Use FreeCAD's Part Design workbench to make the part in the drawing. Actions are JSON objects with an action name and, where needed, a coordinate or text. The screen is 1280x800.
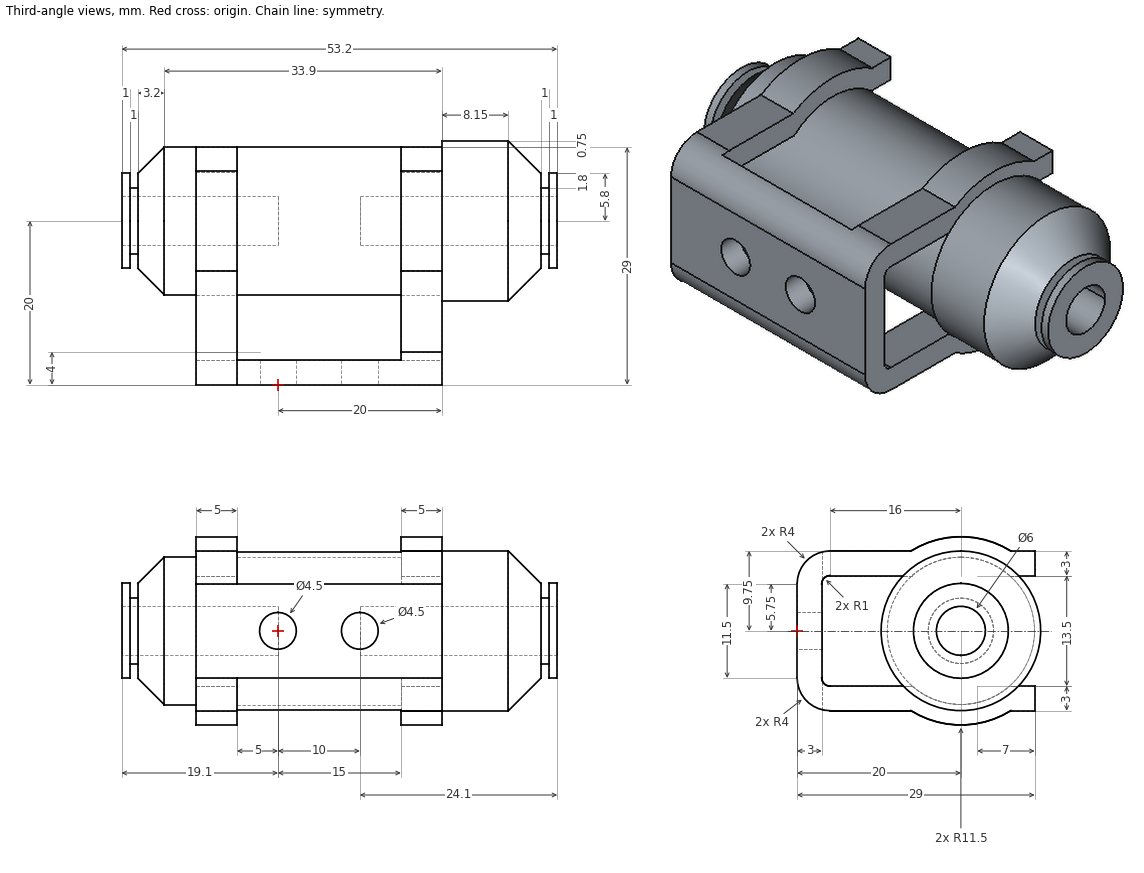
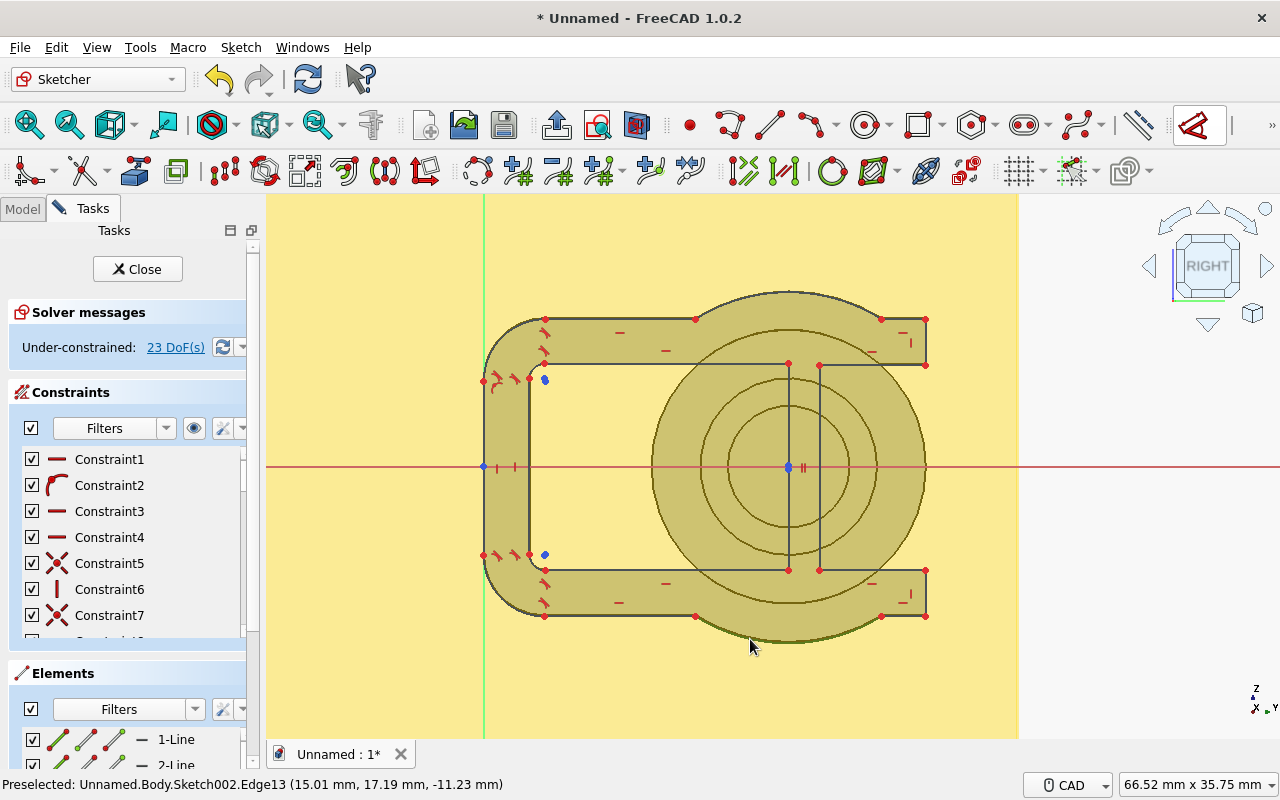
{"action": "left_click", "coordinate": [827, 297]}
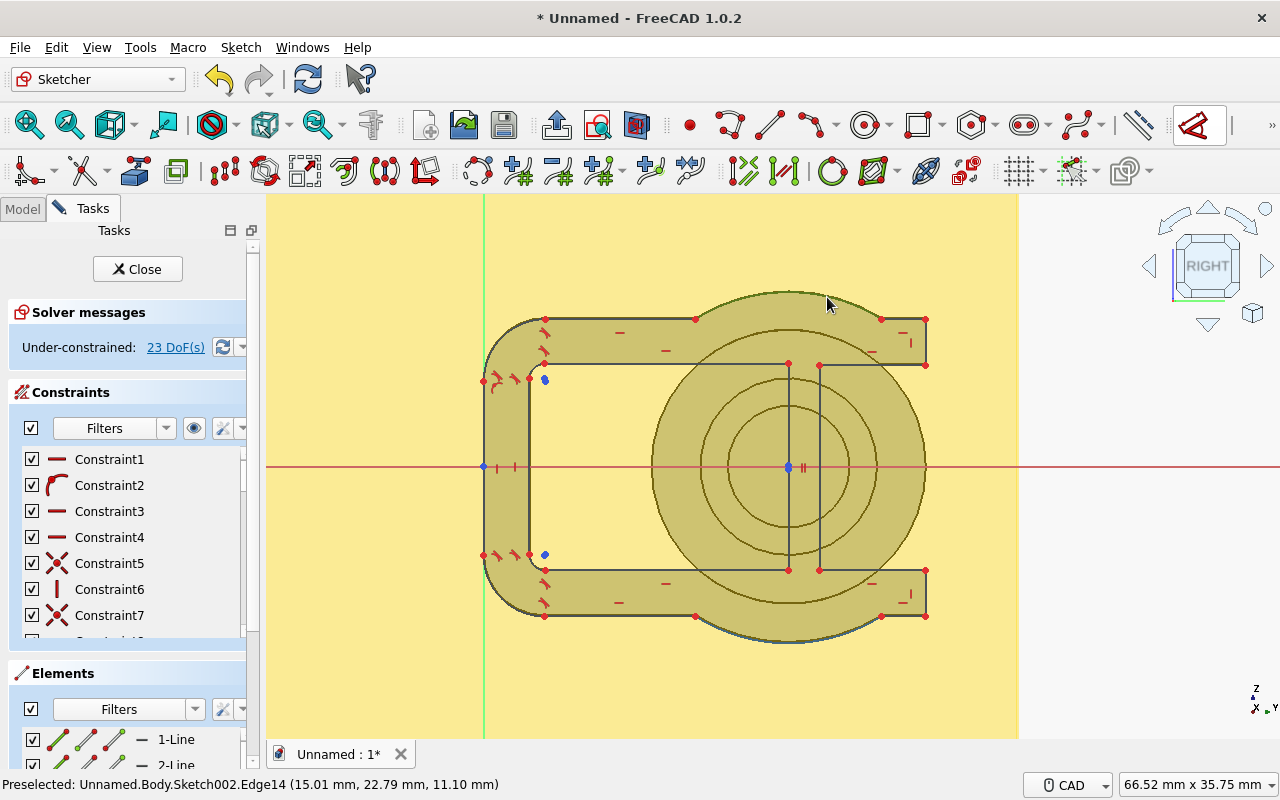
{"action": "key", "text": "c"}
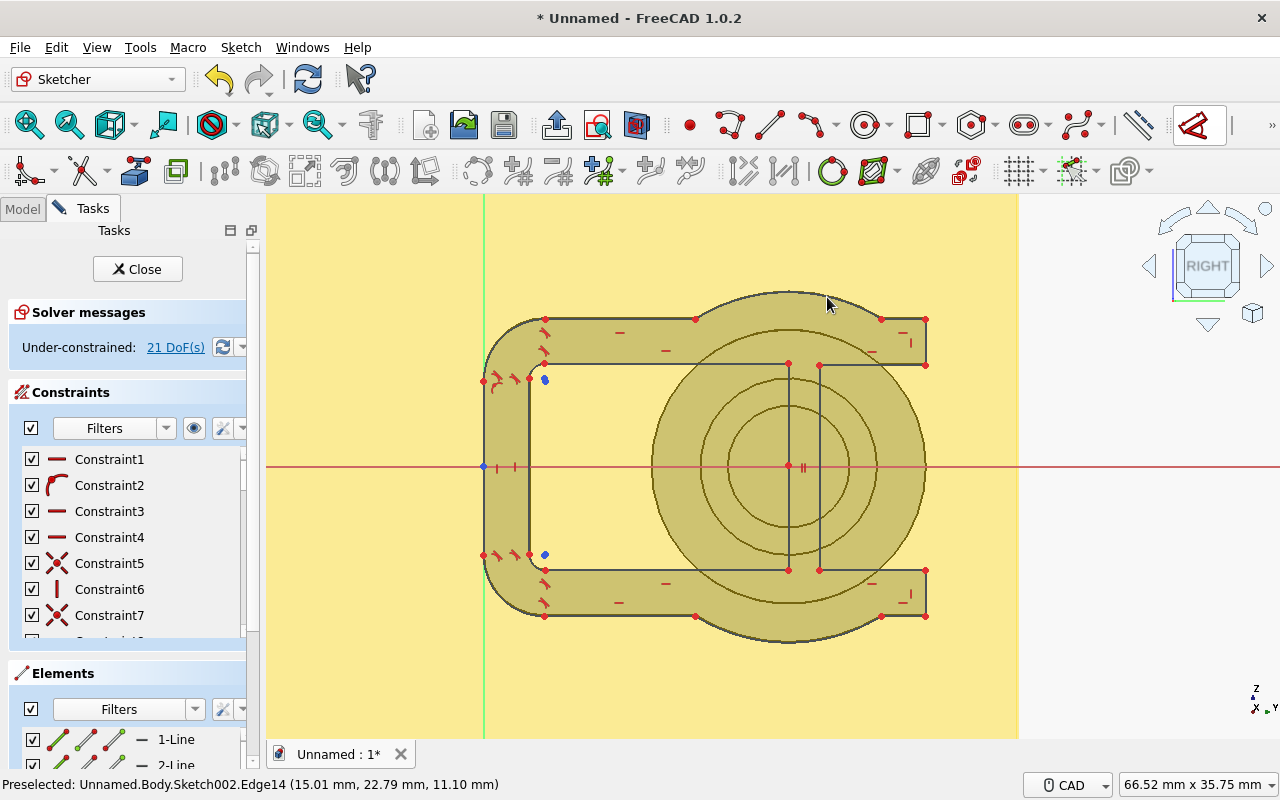
{"action": "left_click", "coordinate": [518, 326]}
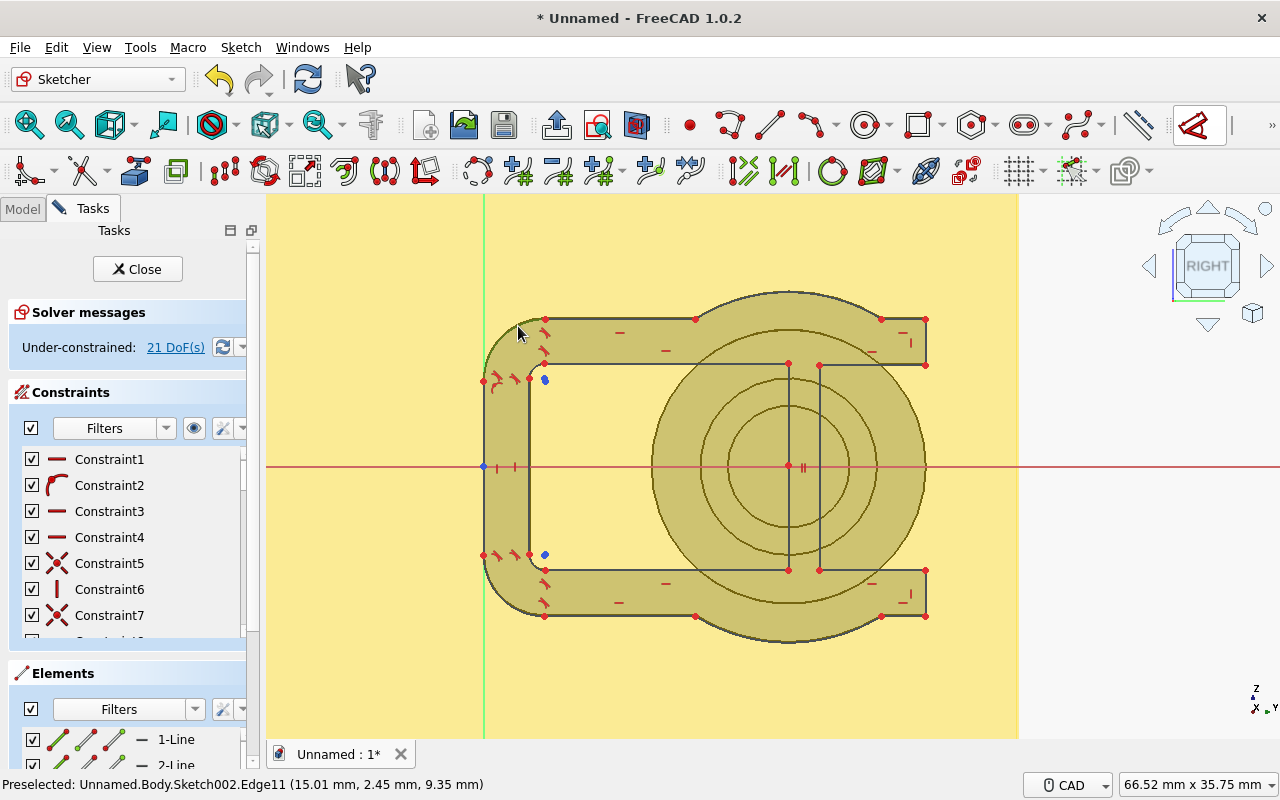
{"action": "left_click", "coordinate": [534, 368]}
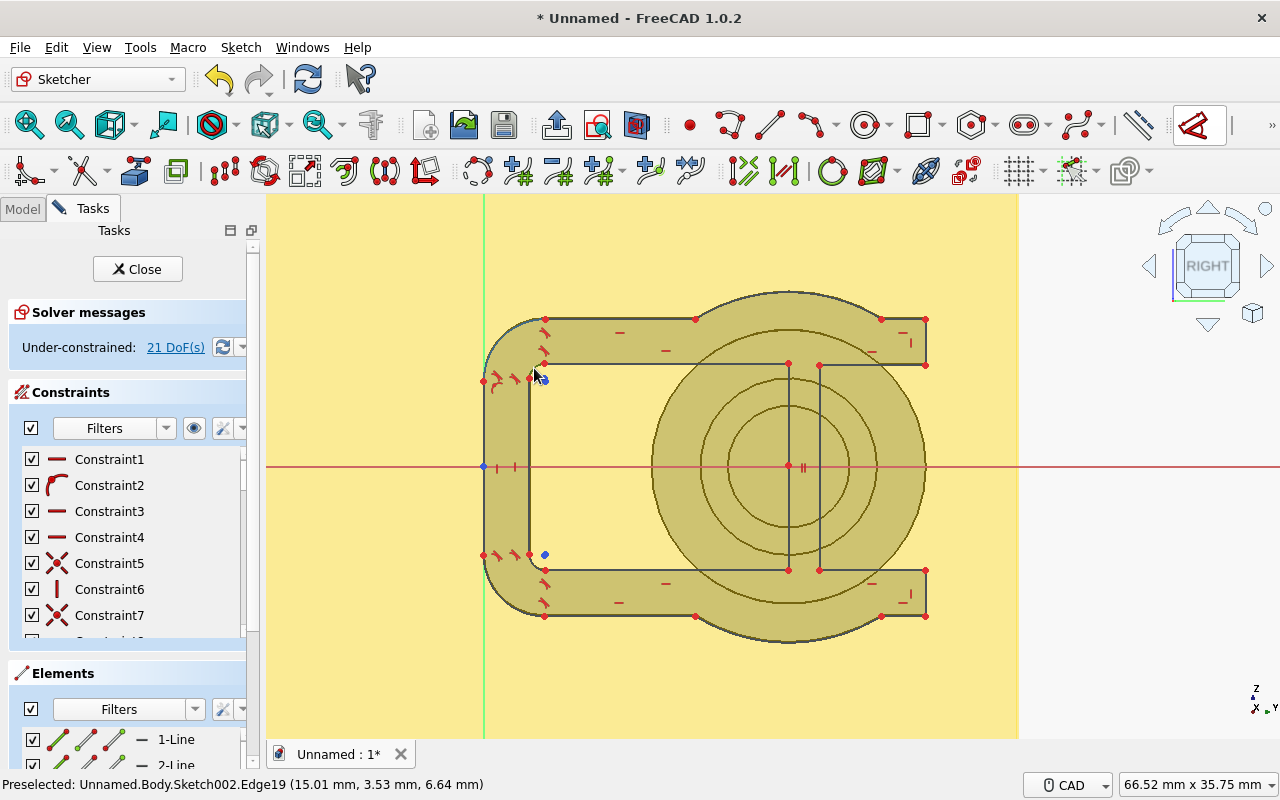
{"action": "key", "text": "c"}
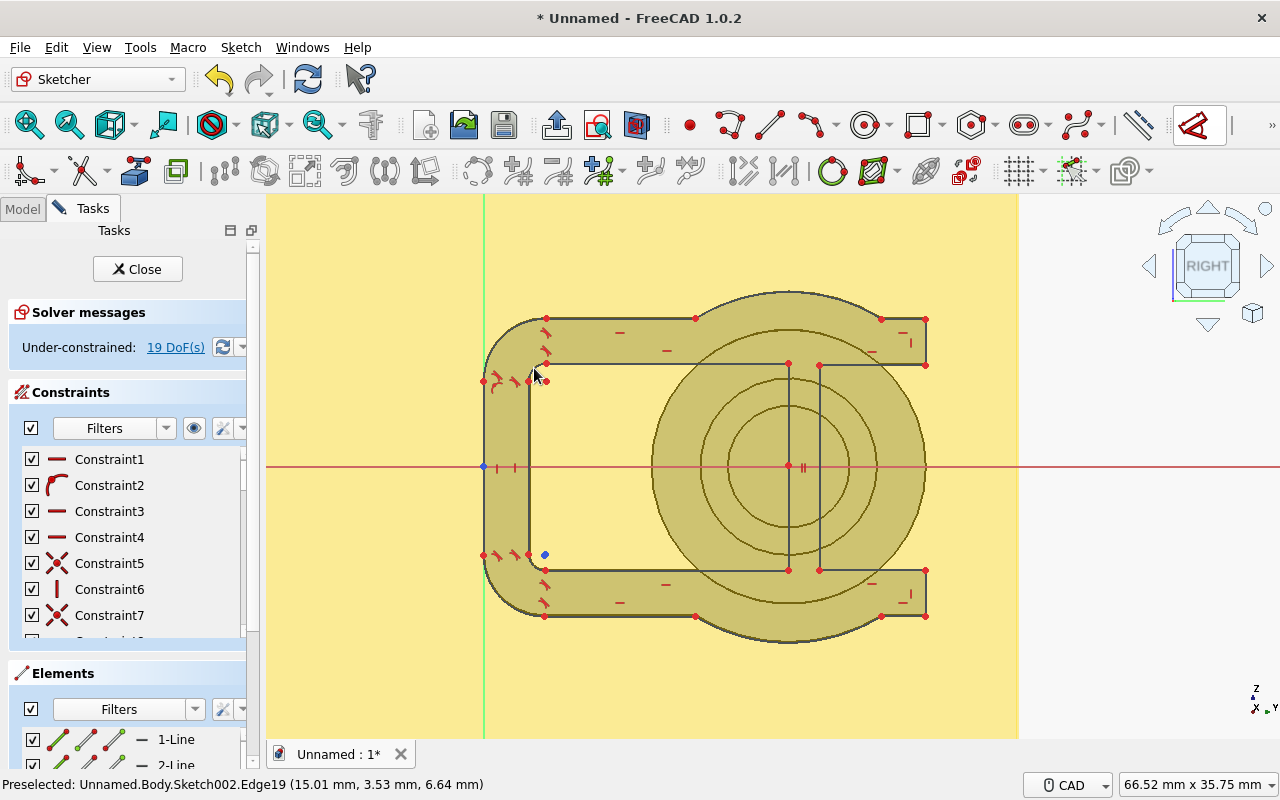
{"action": "left_click", "coordinate": [517, 610]}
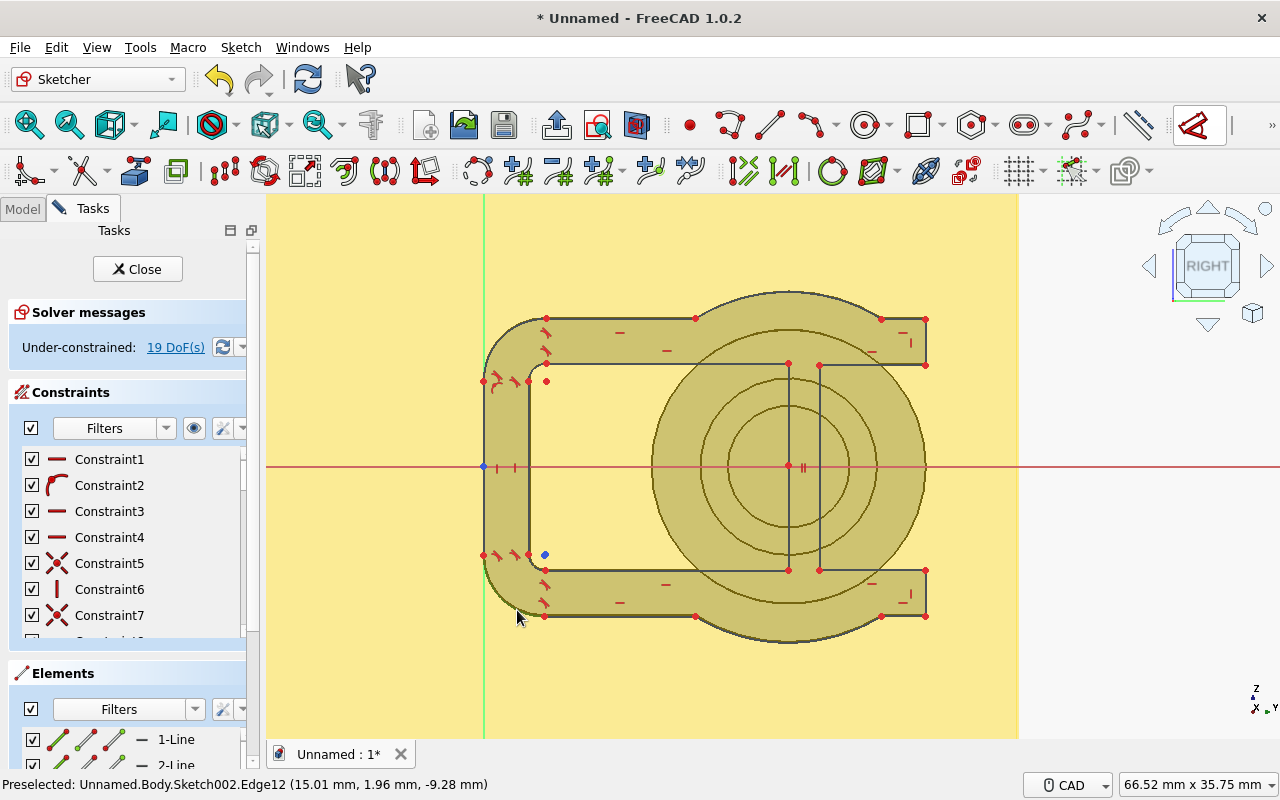
{"action": "left_click", "coordinate": [534, 566]}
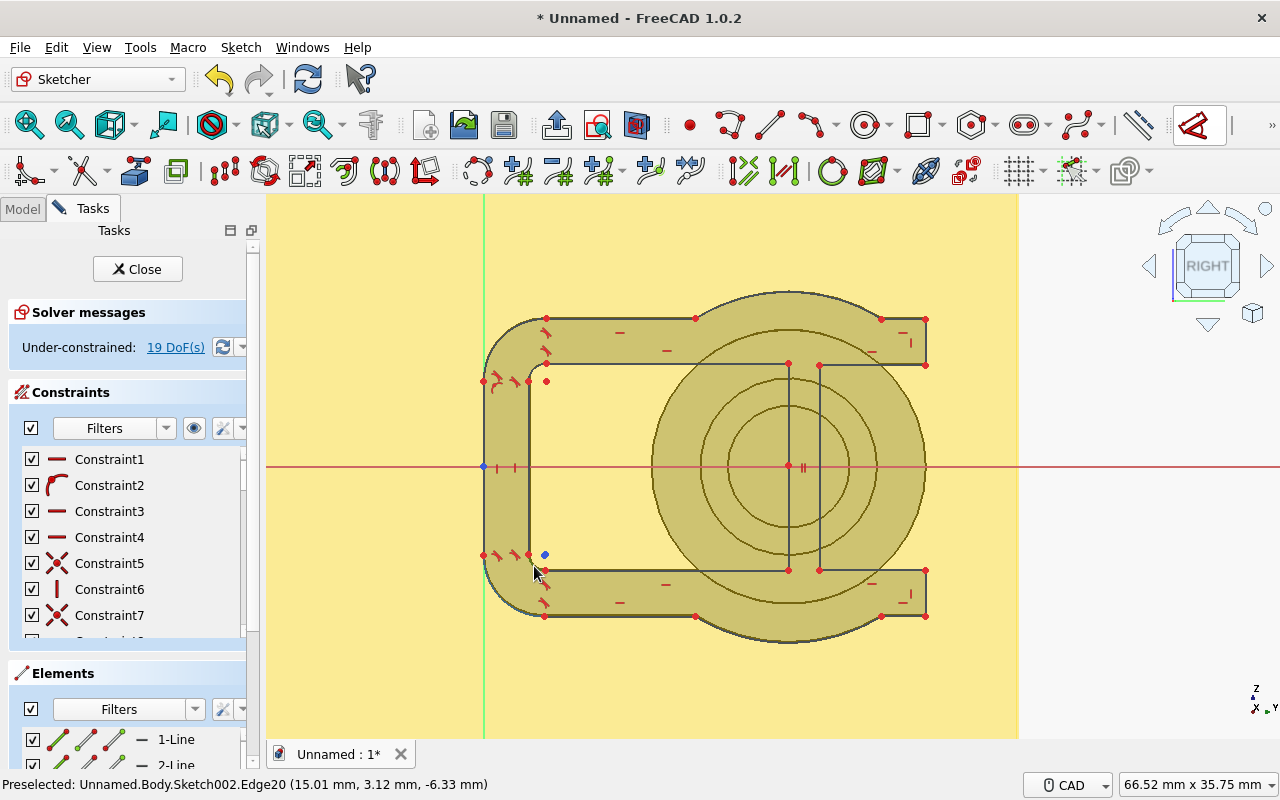
{"action": "key", "text": "c"}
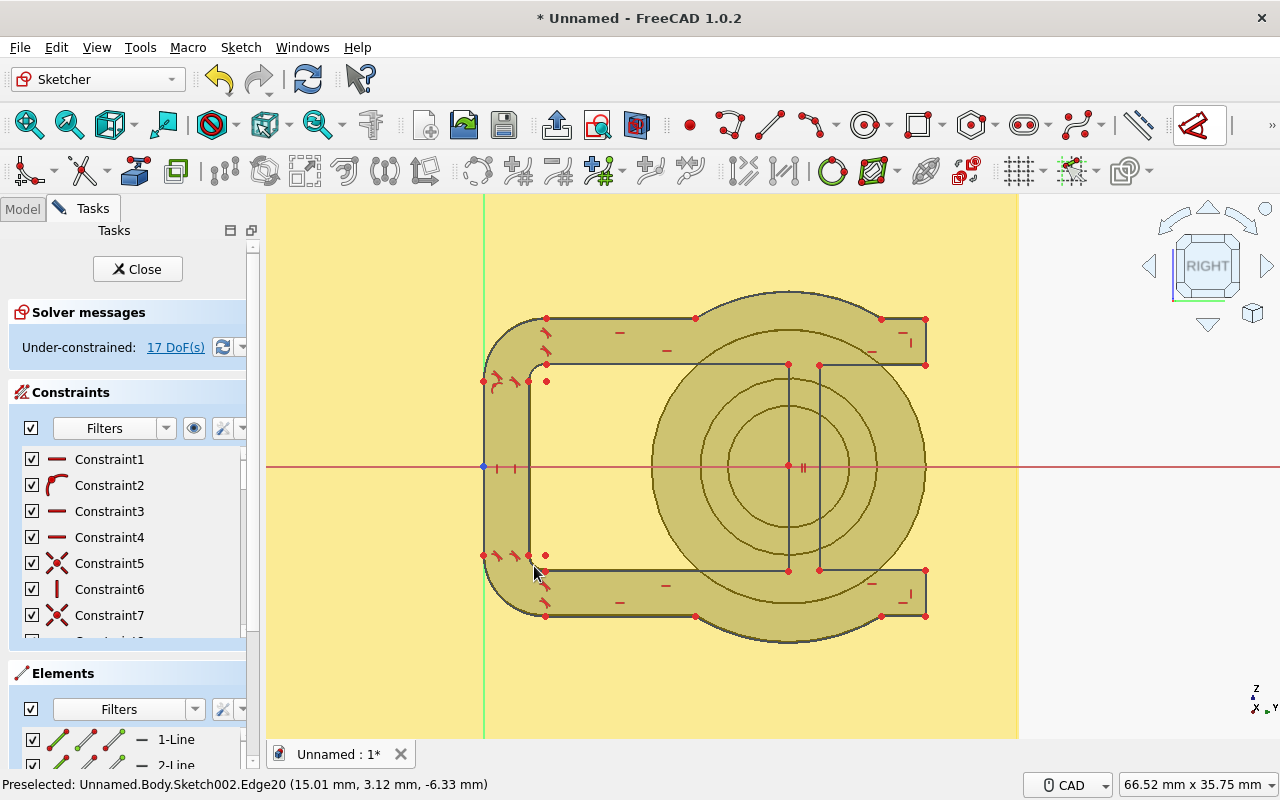
{"action": "left_click", "coordinate": [518, 326]}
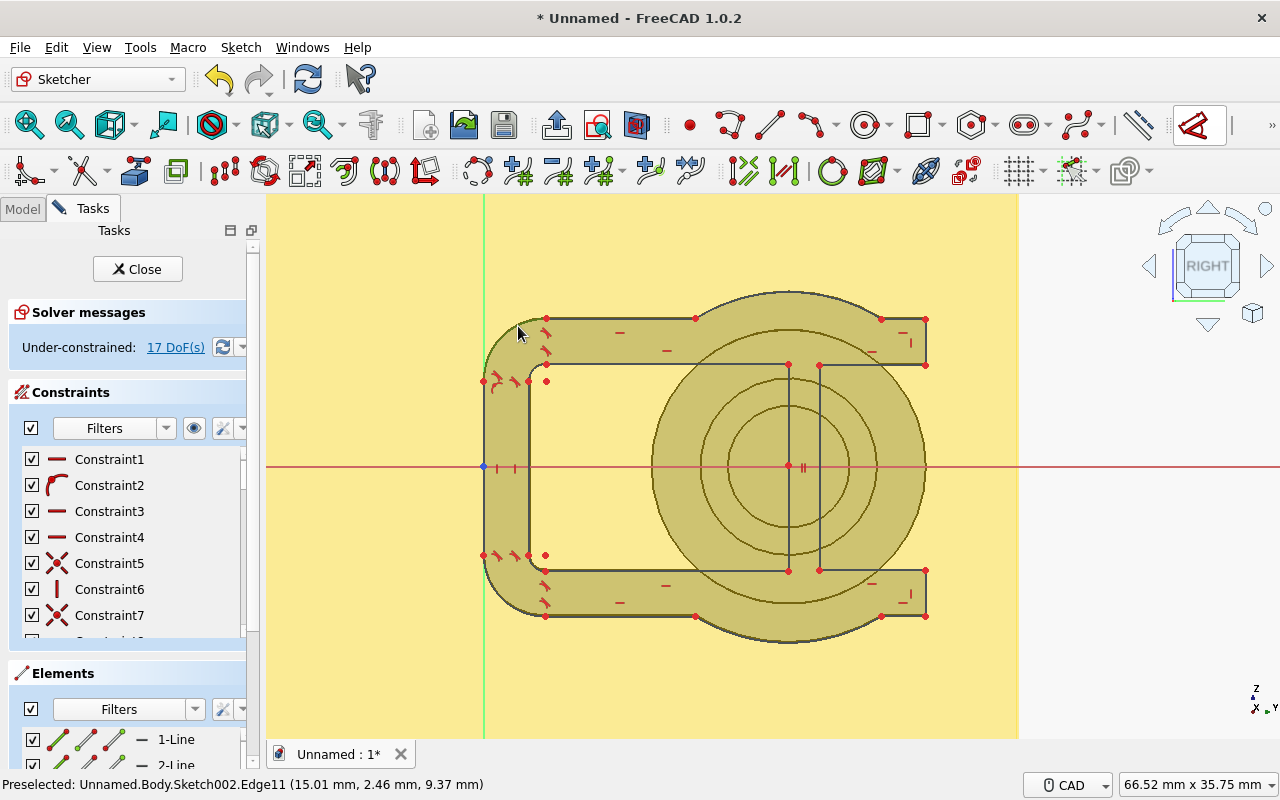
{"action": "left_click", "coordinate": [517, 610]}